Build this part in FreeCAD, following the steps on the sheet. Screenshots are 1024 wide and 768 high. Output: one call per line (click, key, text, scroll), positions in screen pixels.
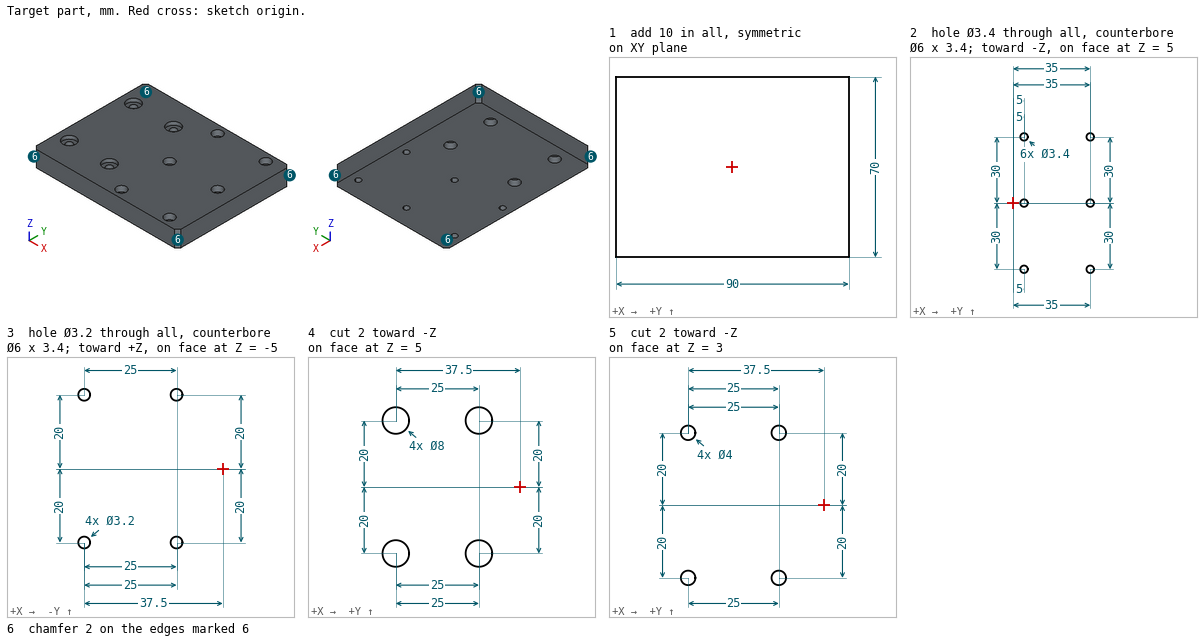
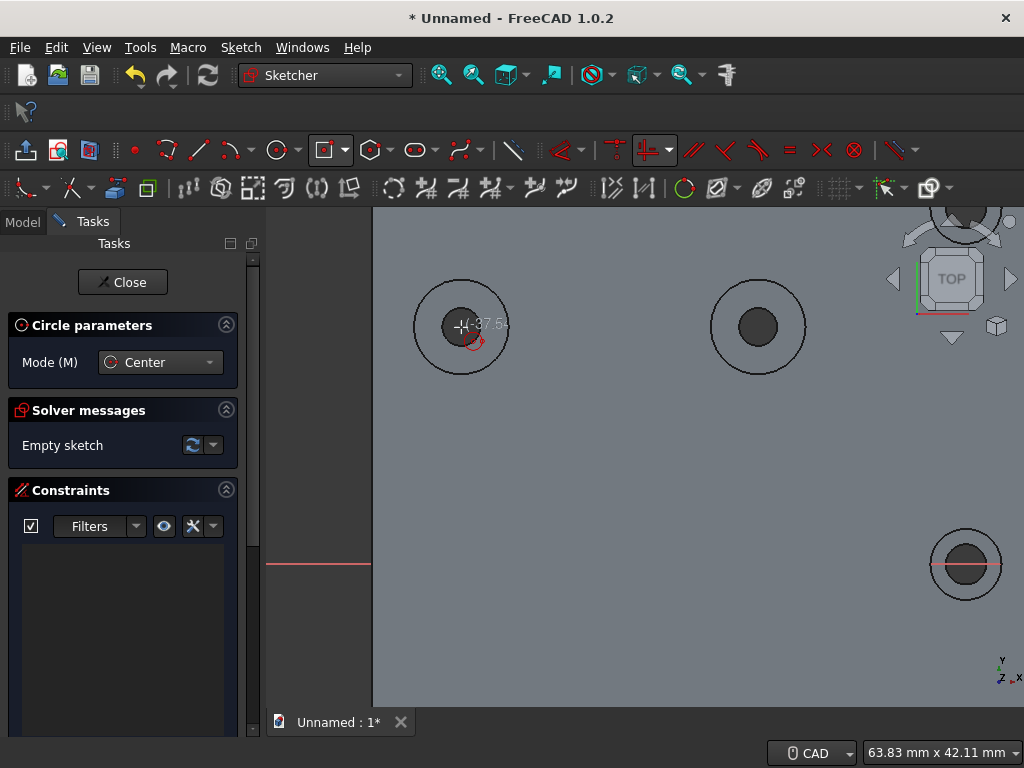
click(461, 327)
click(478, 310)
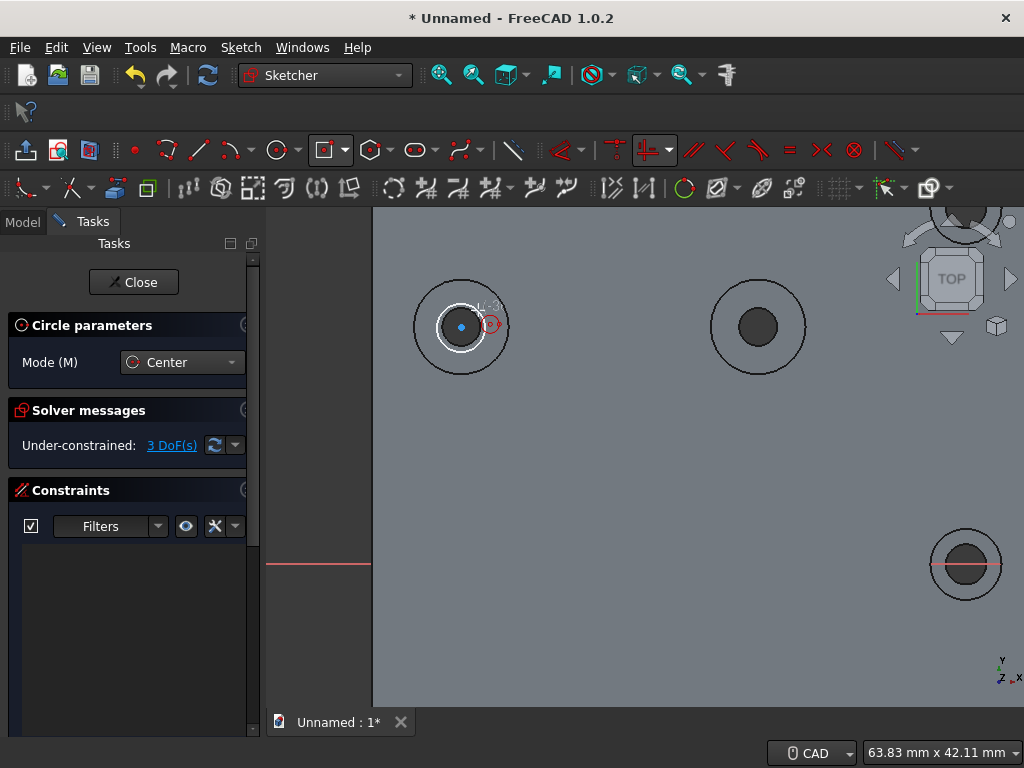
scroll(460, 326, down, 3)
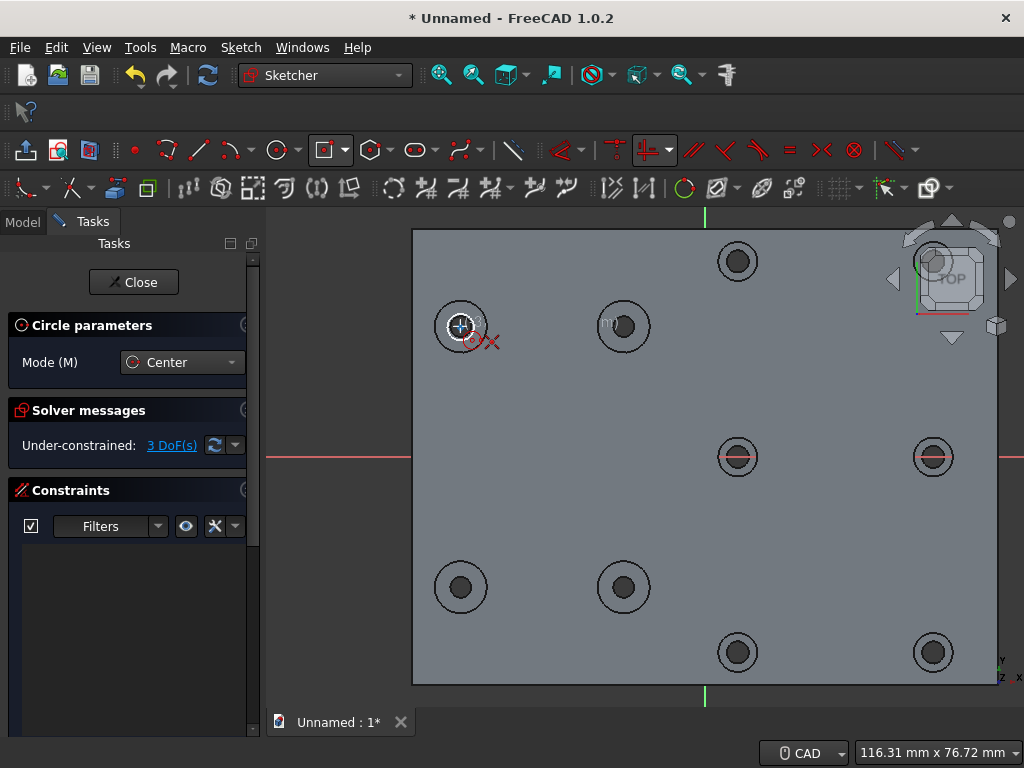
scroll(461, 587, up, 3)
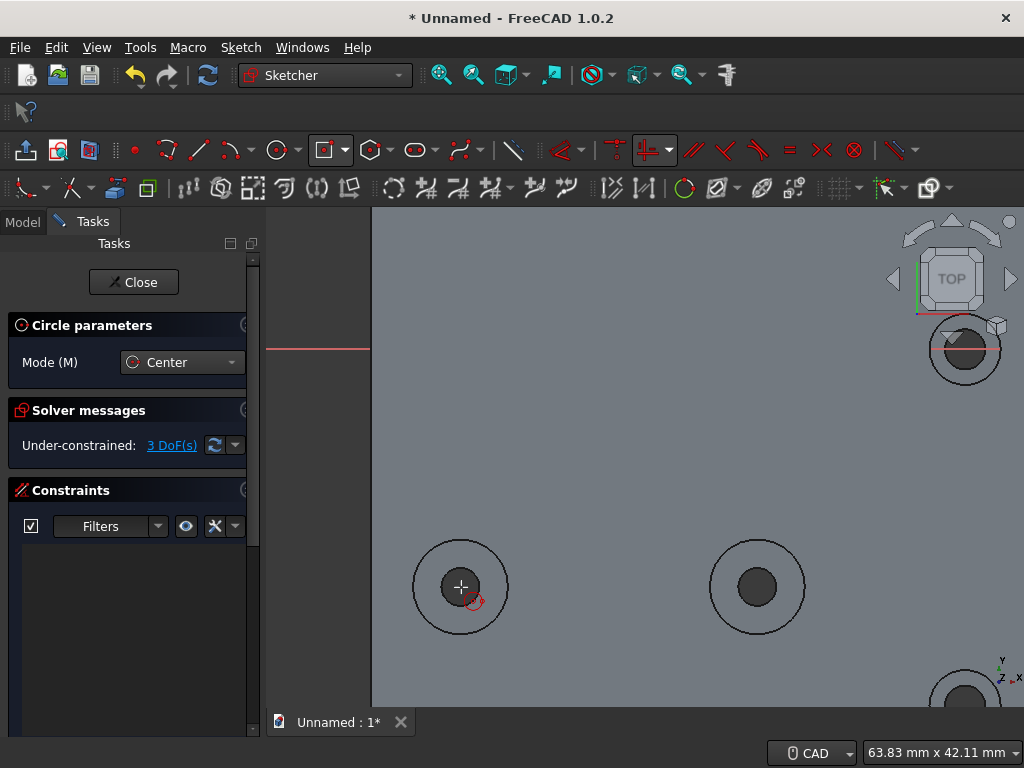
click(460, 587)
click(477, 570)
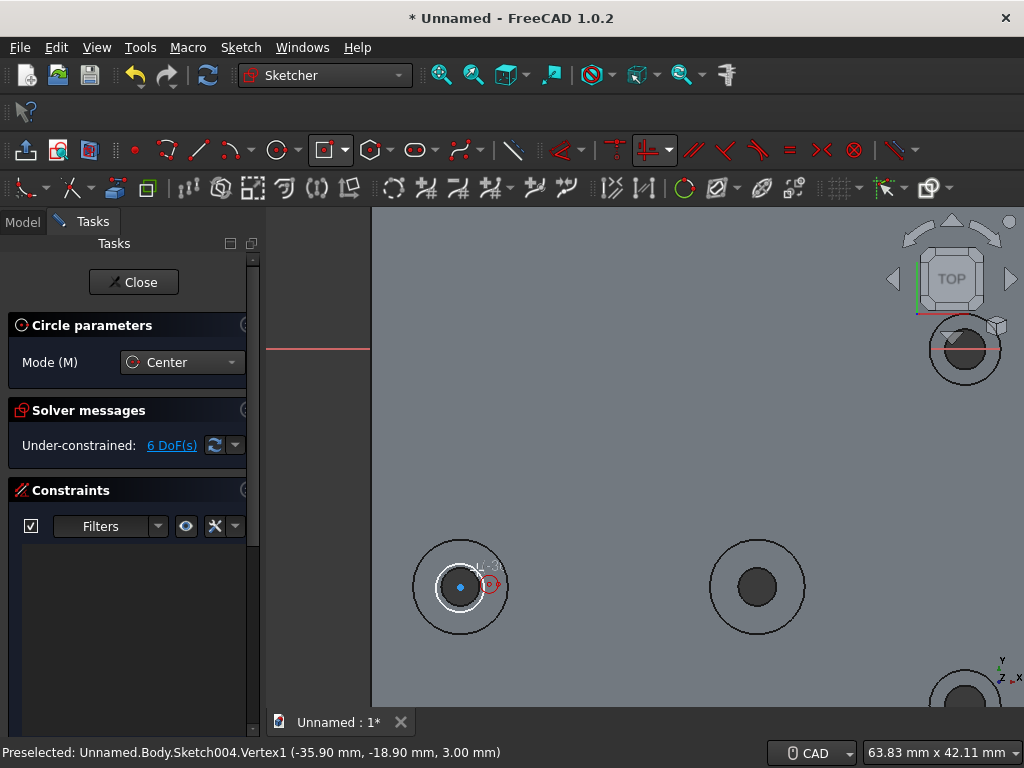
click(757, 587)
click(774, 570)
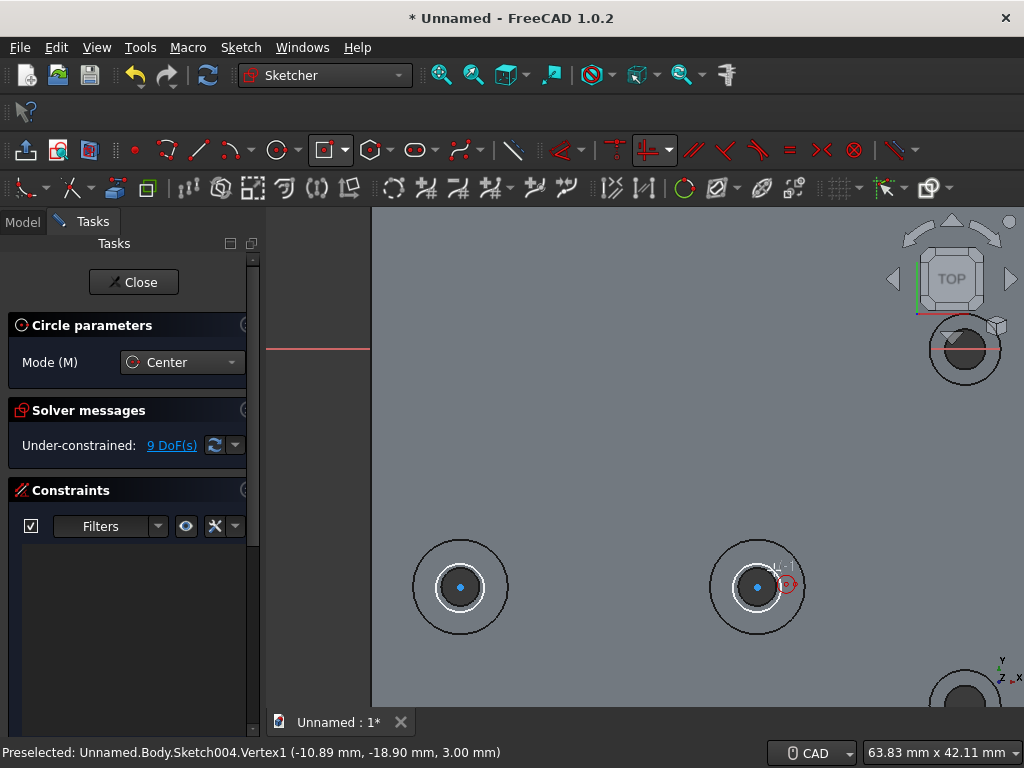
scroll(461, 588, down, 3)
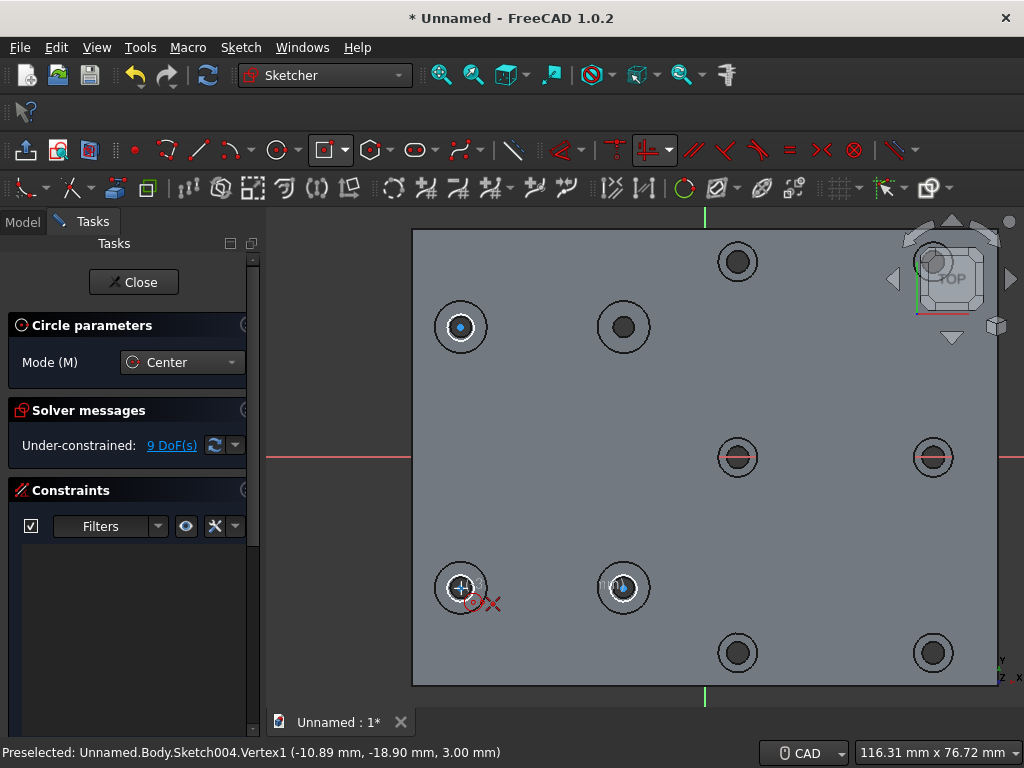
scroll(624, 327, up, 3)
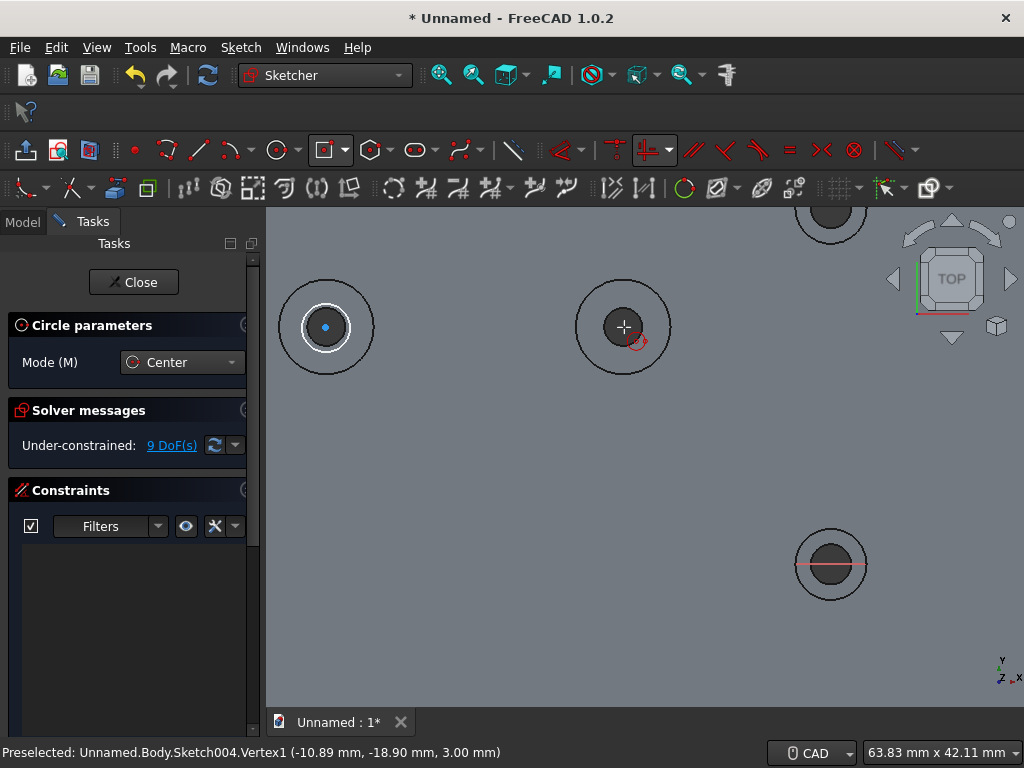
click(623, 327)
click(640, 310)
key(Escape)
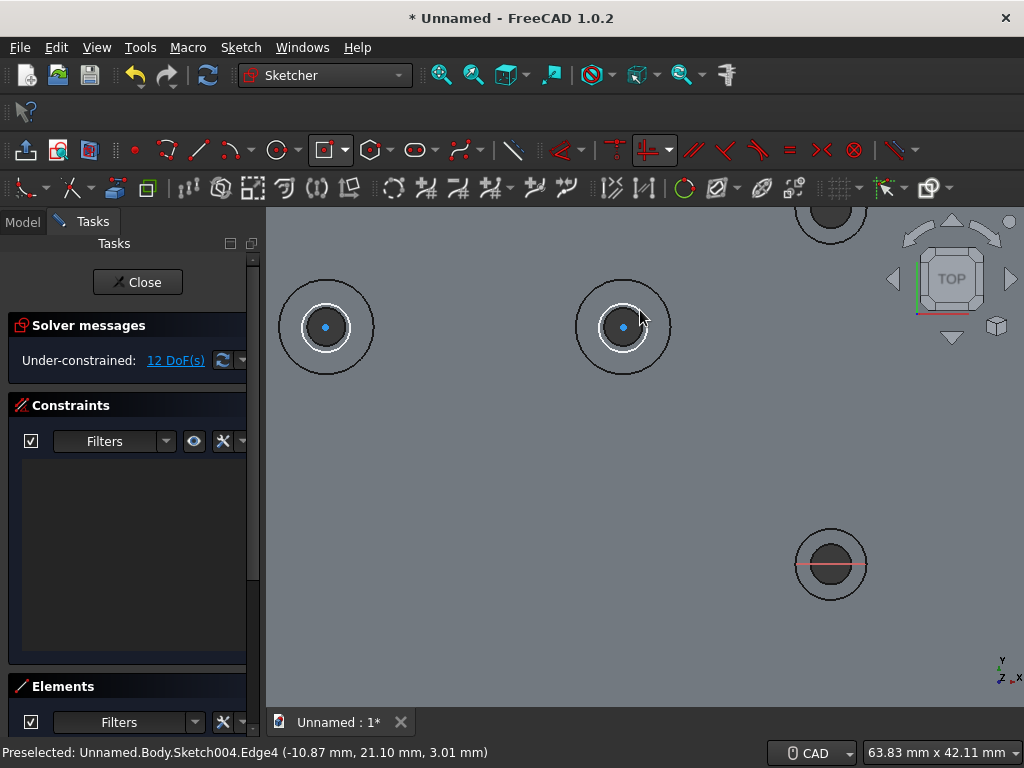
click(343, 311)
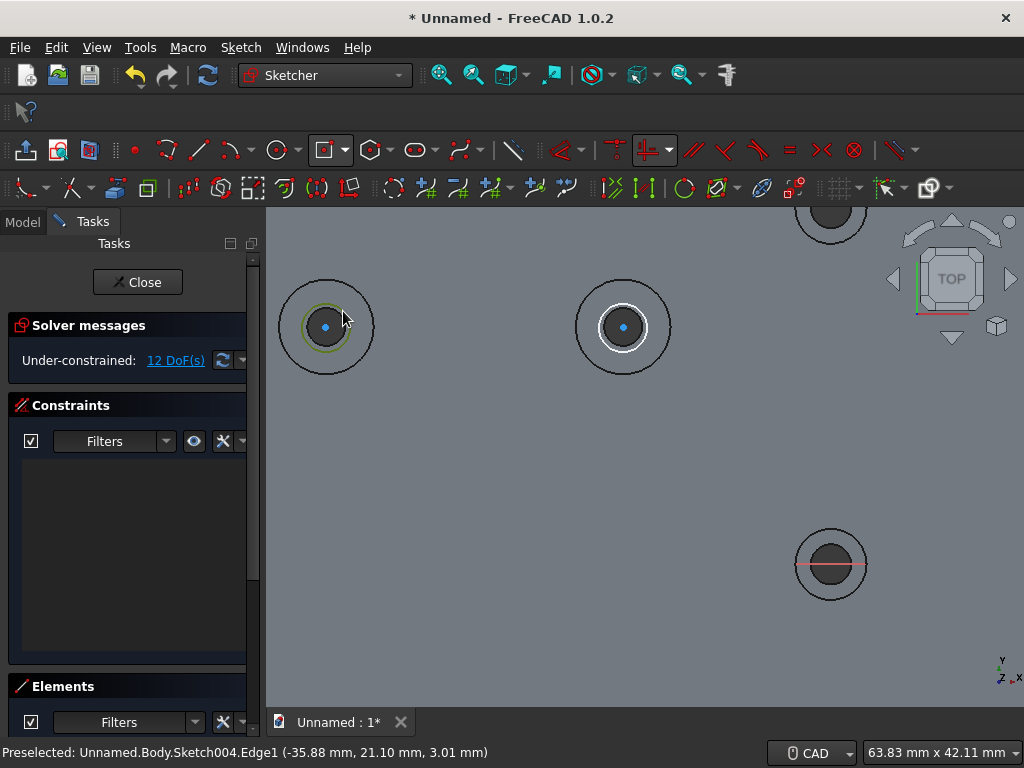
scroll(624, 326, down, 3)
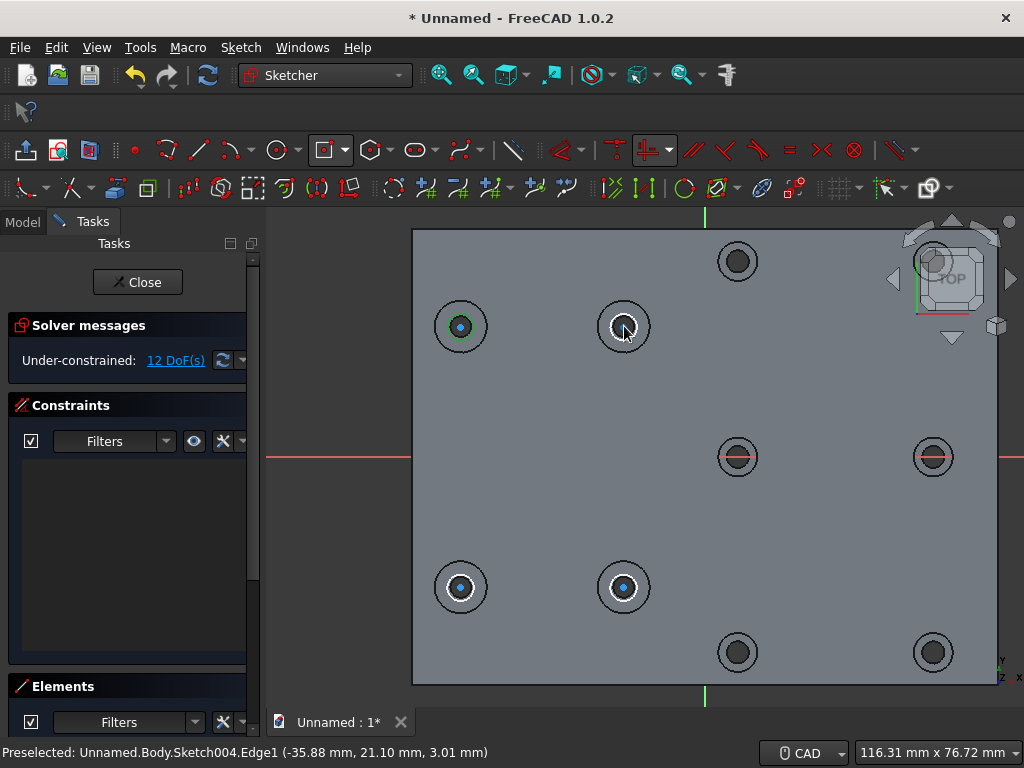
click(470, 579)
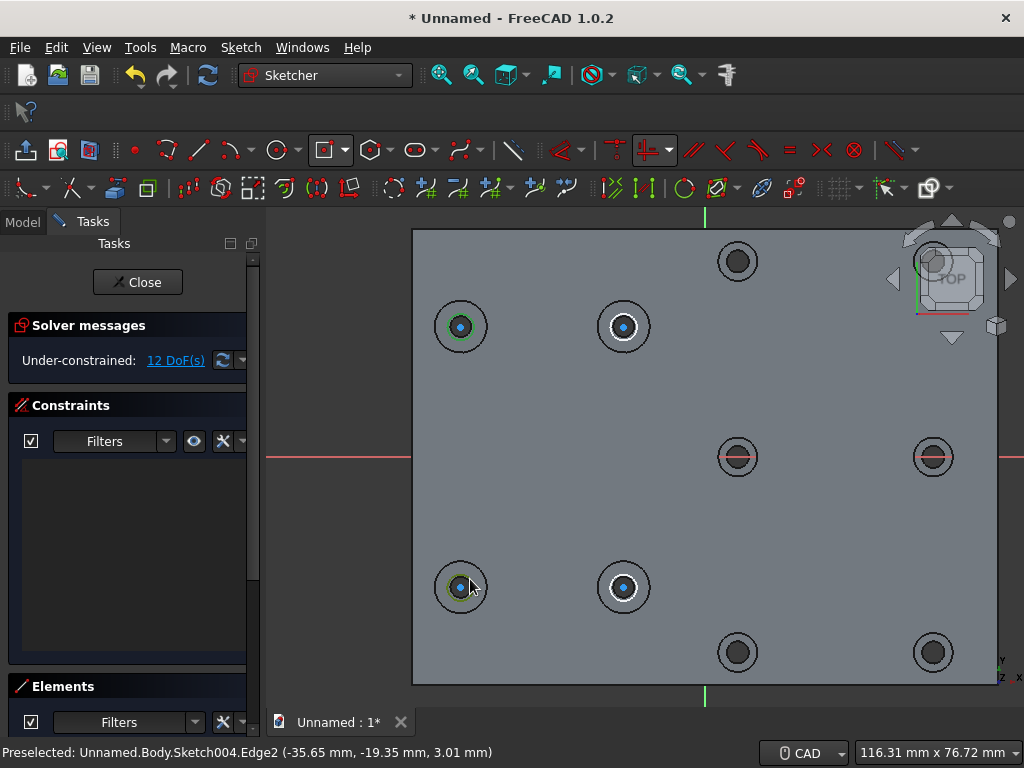
click(633, 579)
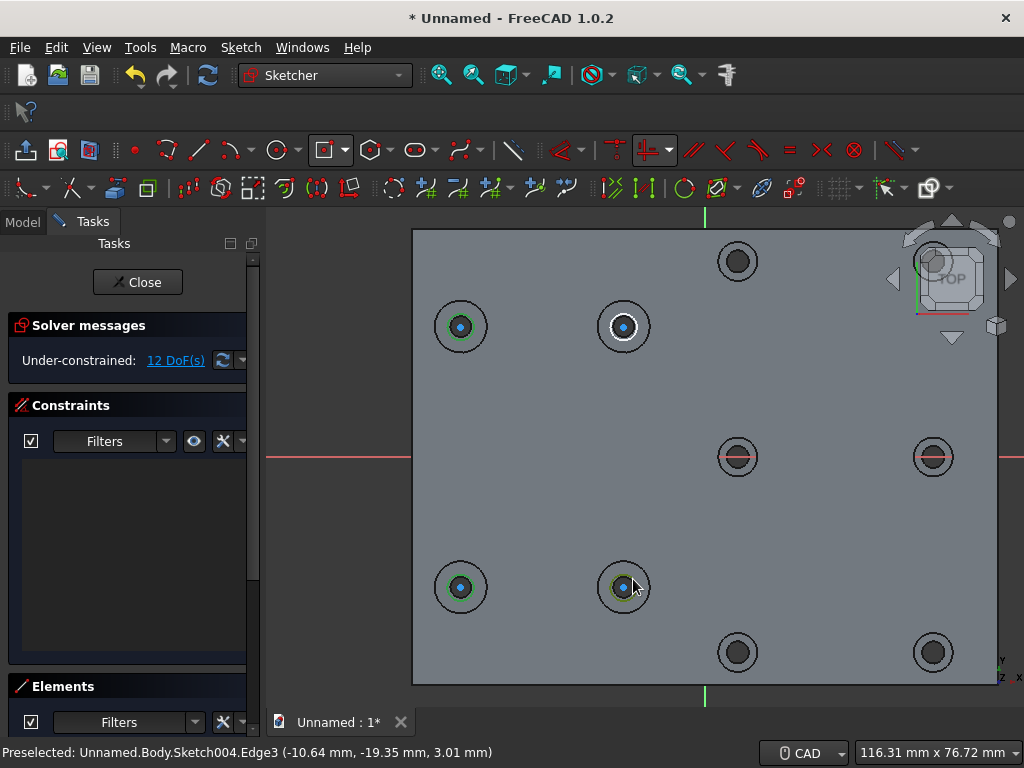
click(633, 318)